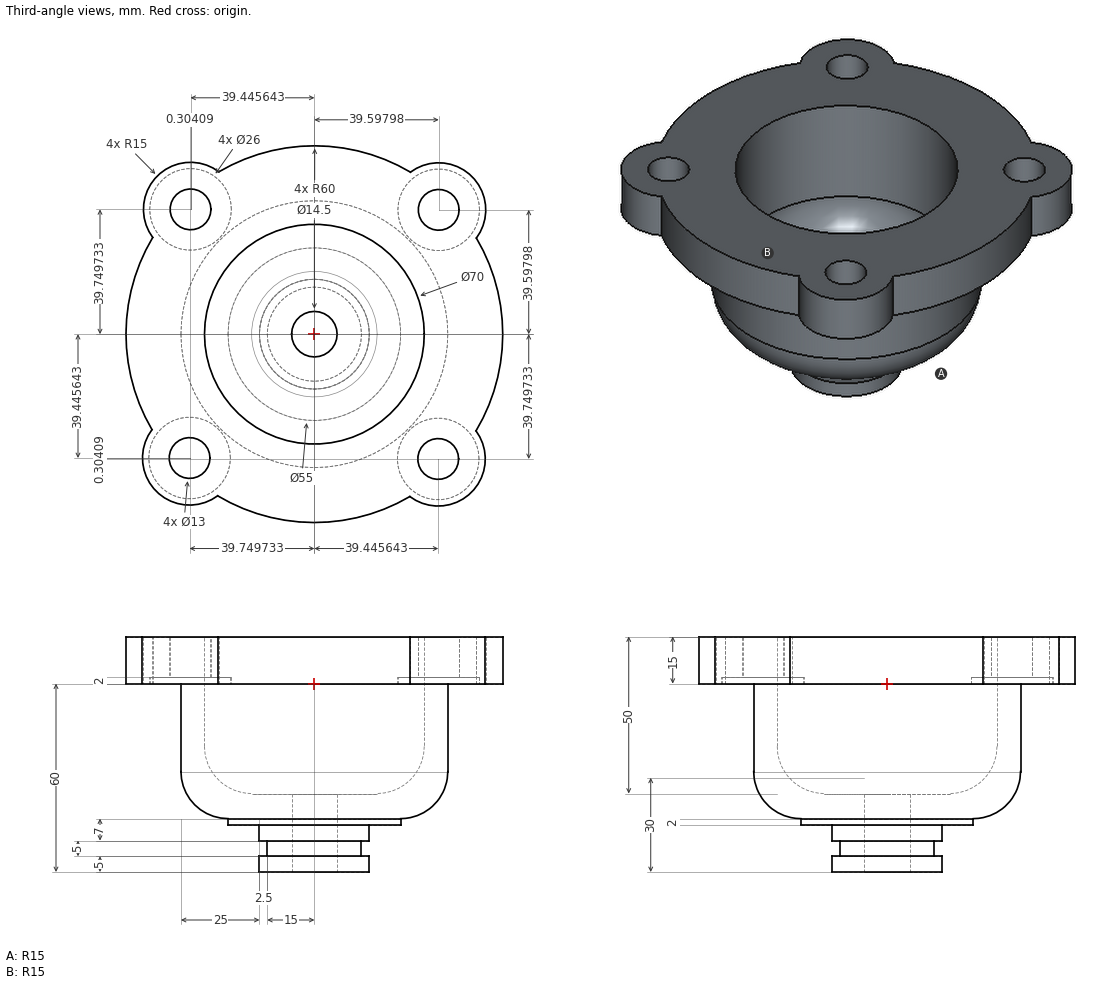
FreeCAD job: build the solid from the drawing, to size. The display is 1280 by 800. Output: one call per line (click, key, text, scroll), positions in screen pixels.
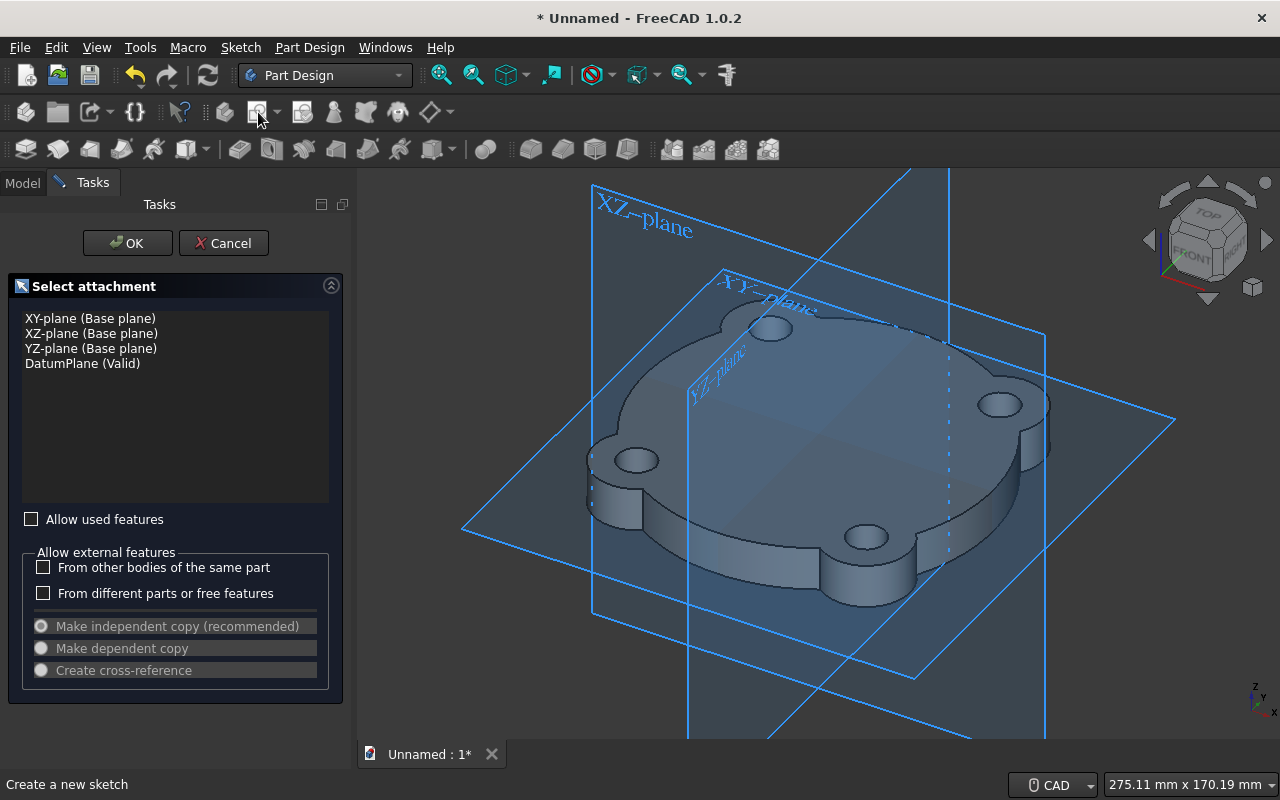
click(82, 334)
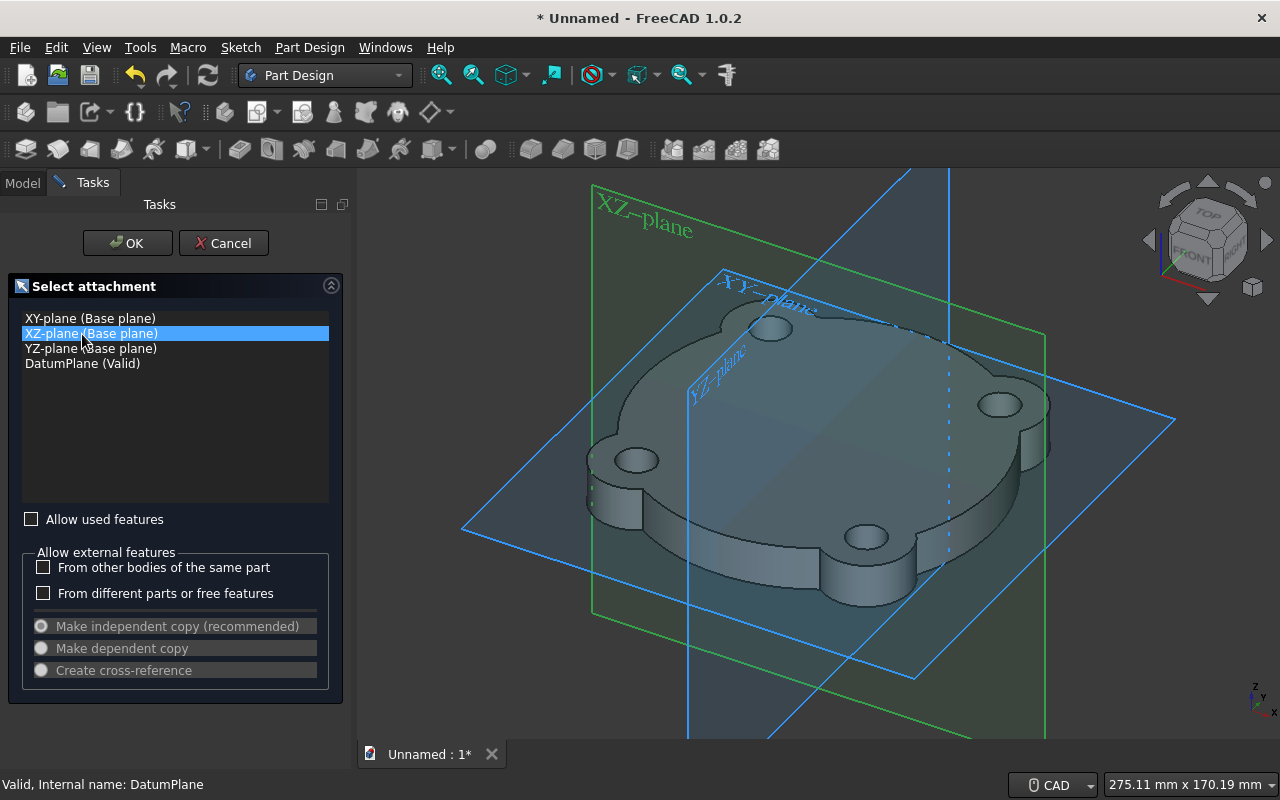
click(128, 243)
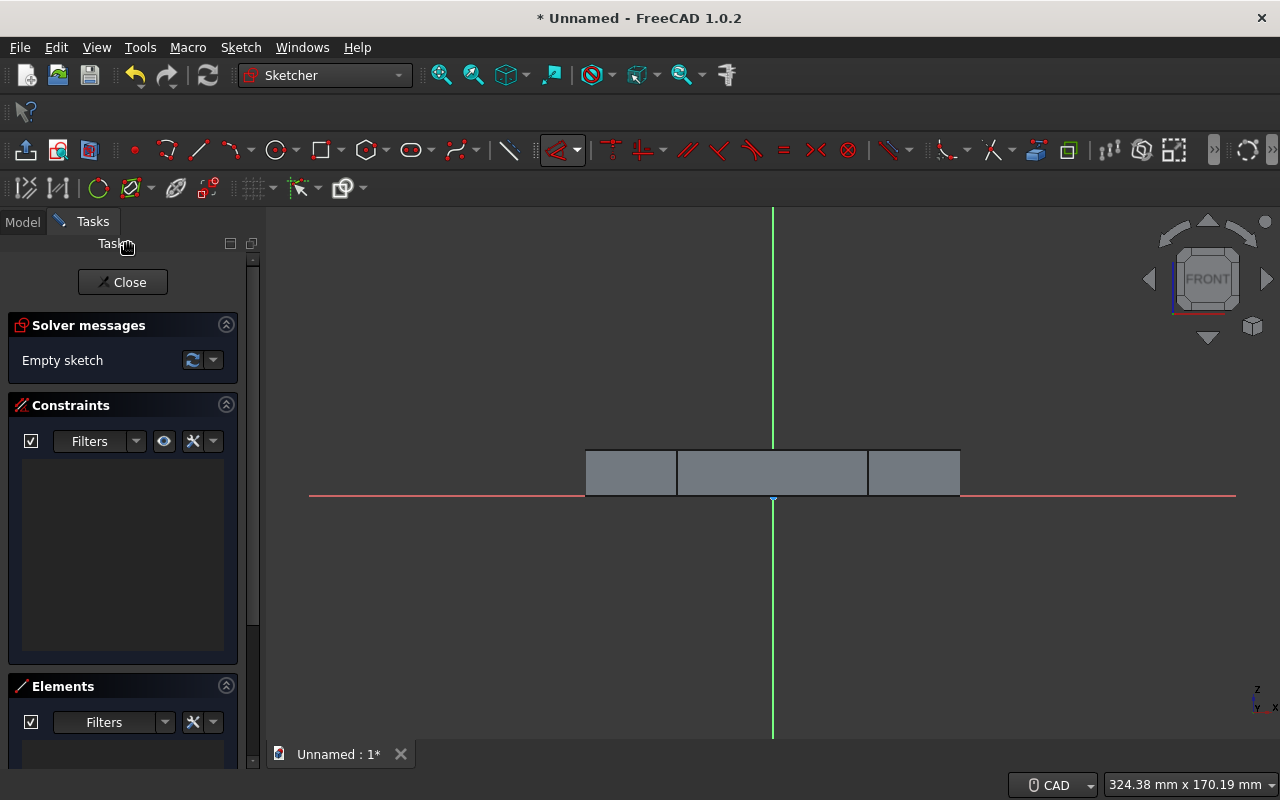
click(90, 150)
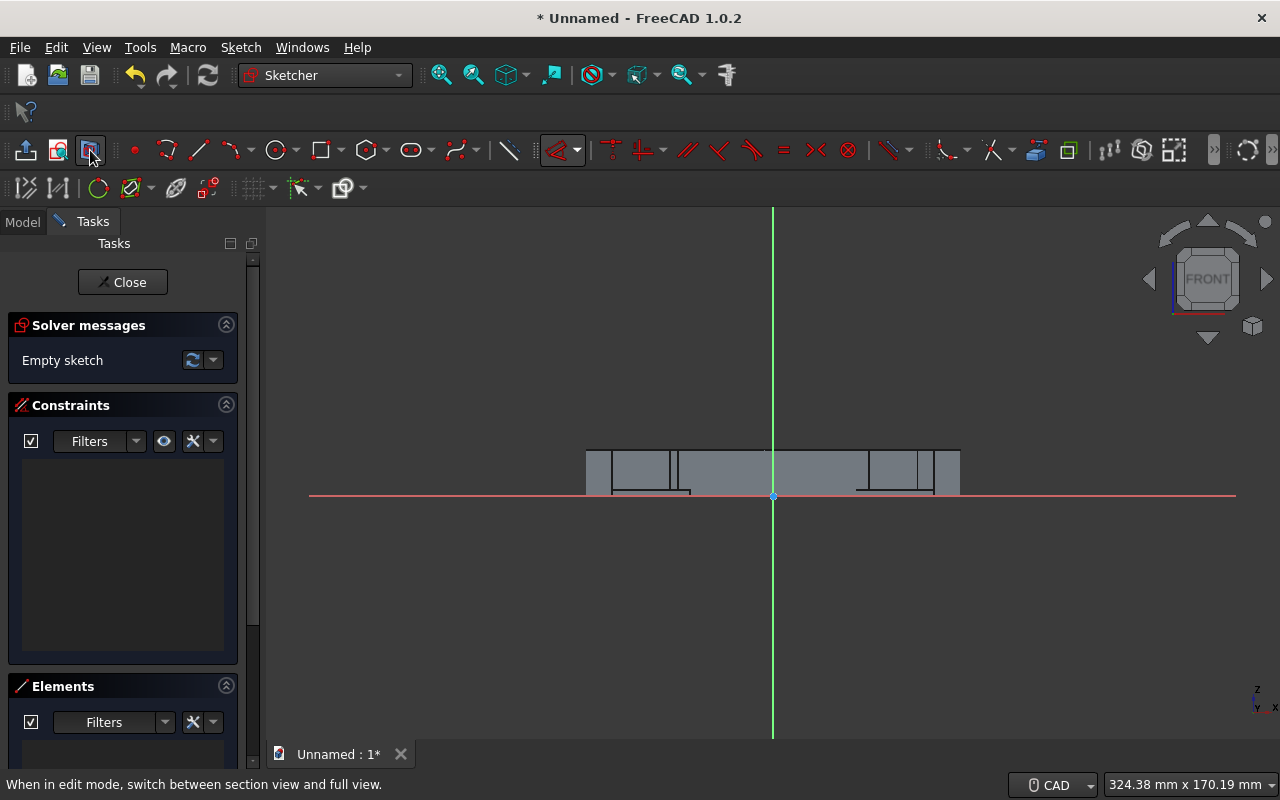
scroll(709, 711, up, 3)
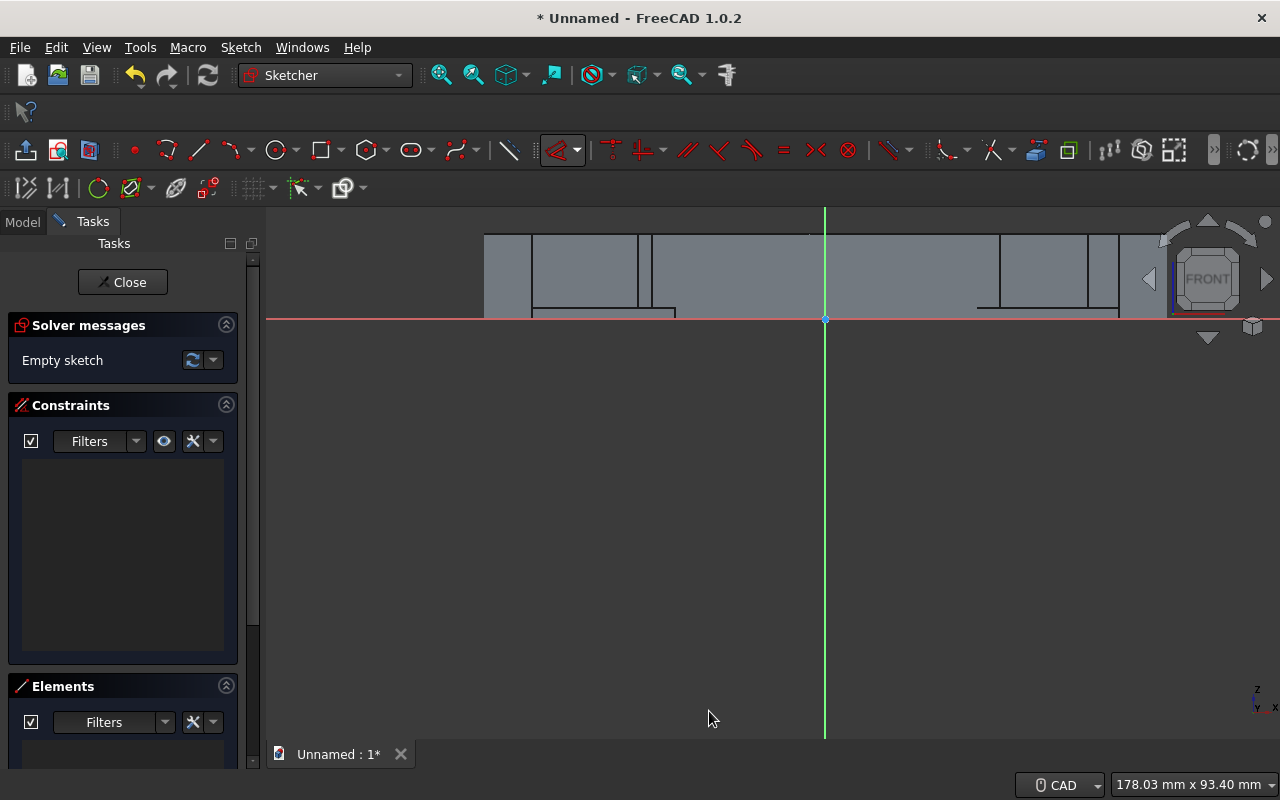
click(168, 150)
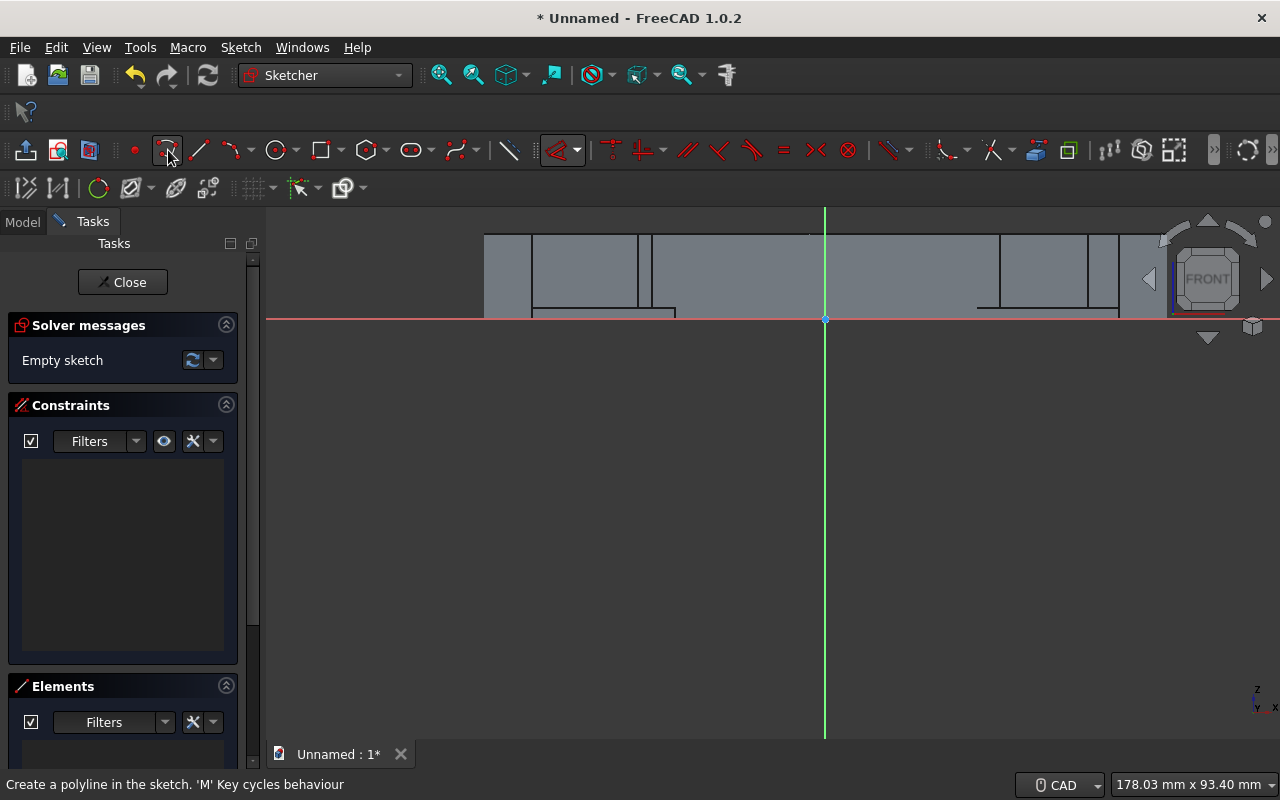
click(825, 319)
click(816, 661)
click(726, 661)
click(726, 633)
click(740, 633)
click(740, 604)
click(726, 604)
click(726, 564)
click(583, 564)
click(583, 328)
click(825, 319)
key(Escape)
key(Escape)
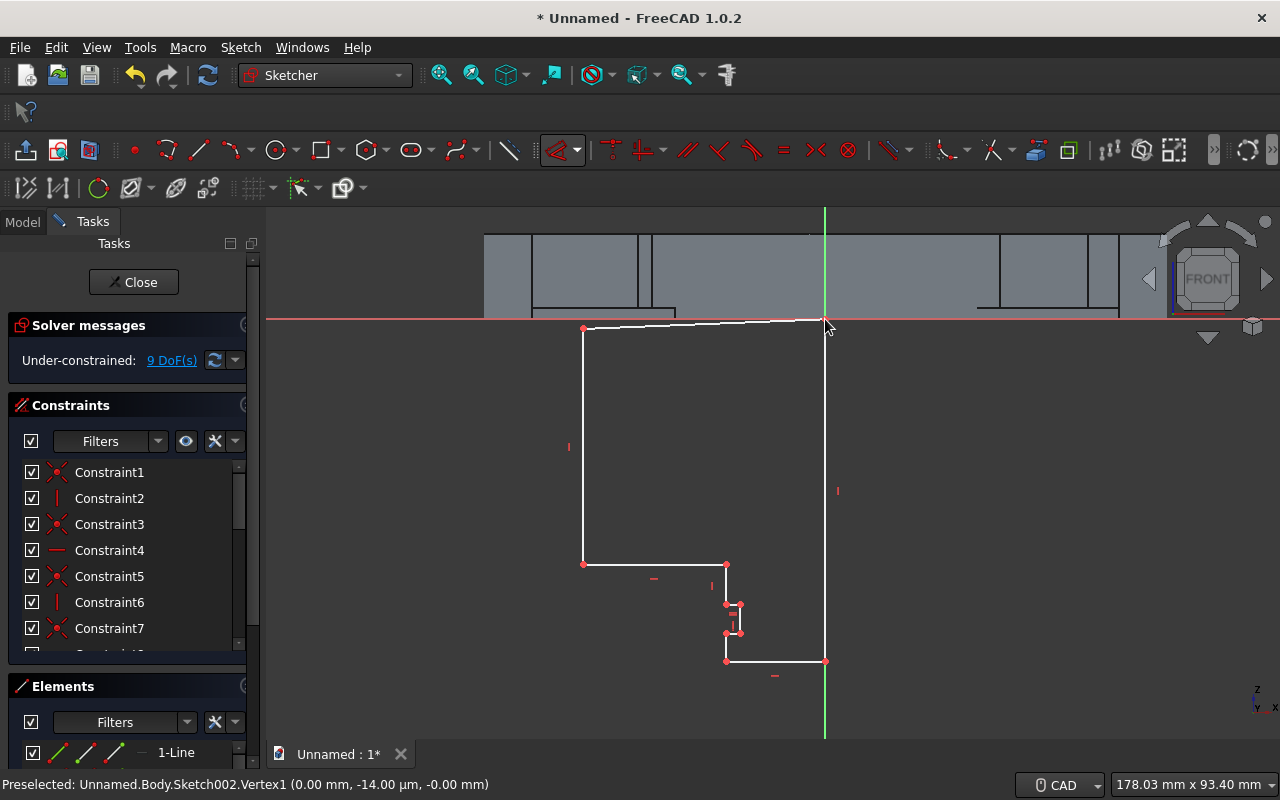
click(753, 322)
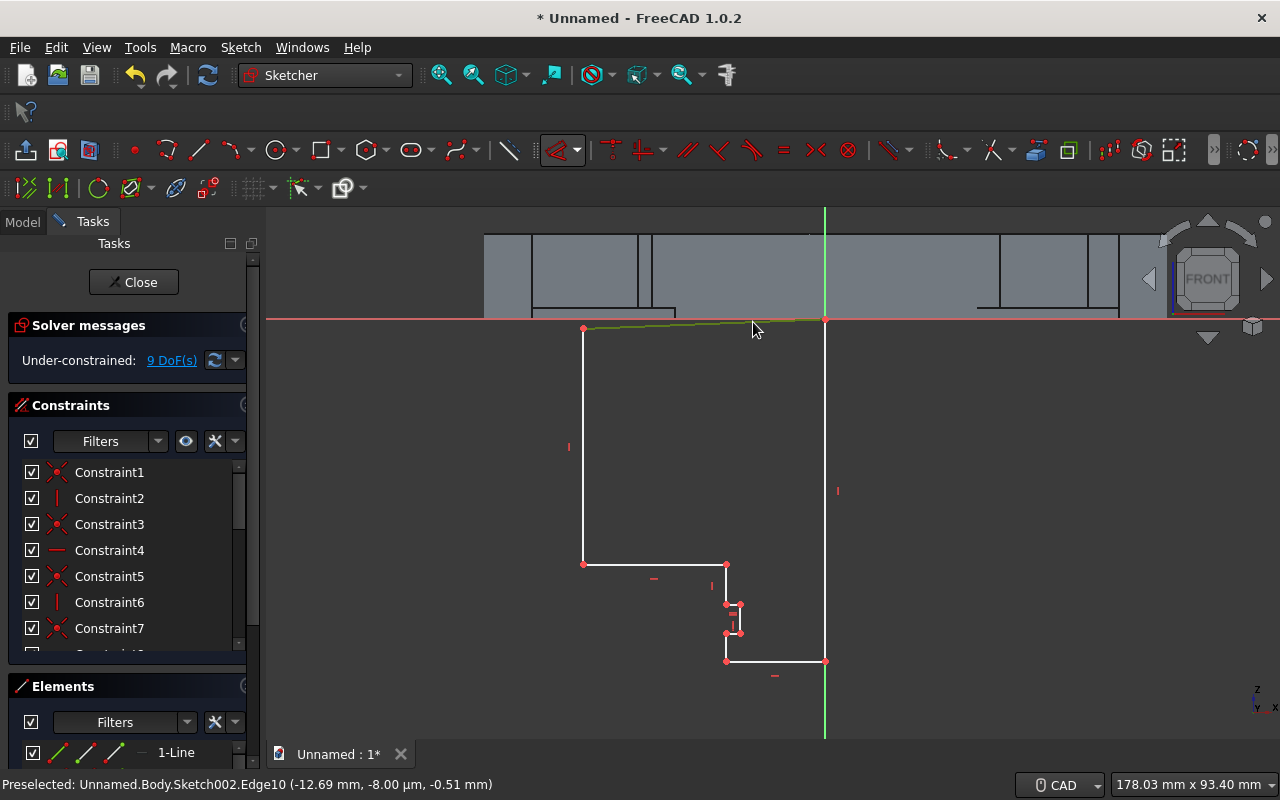
key(h)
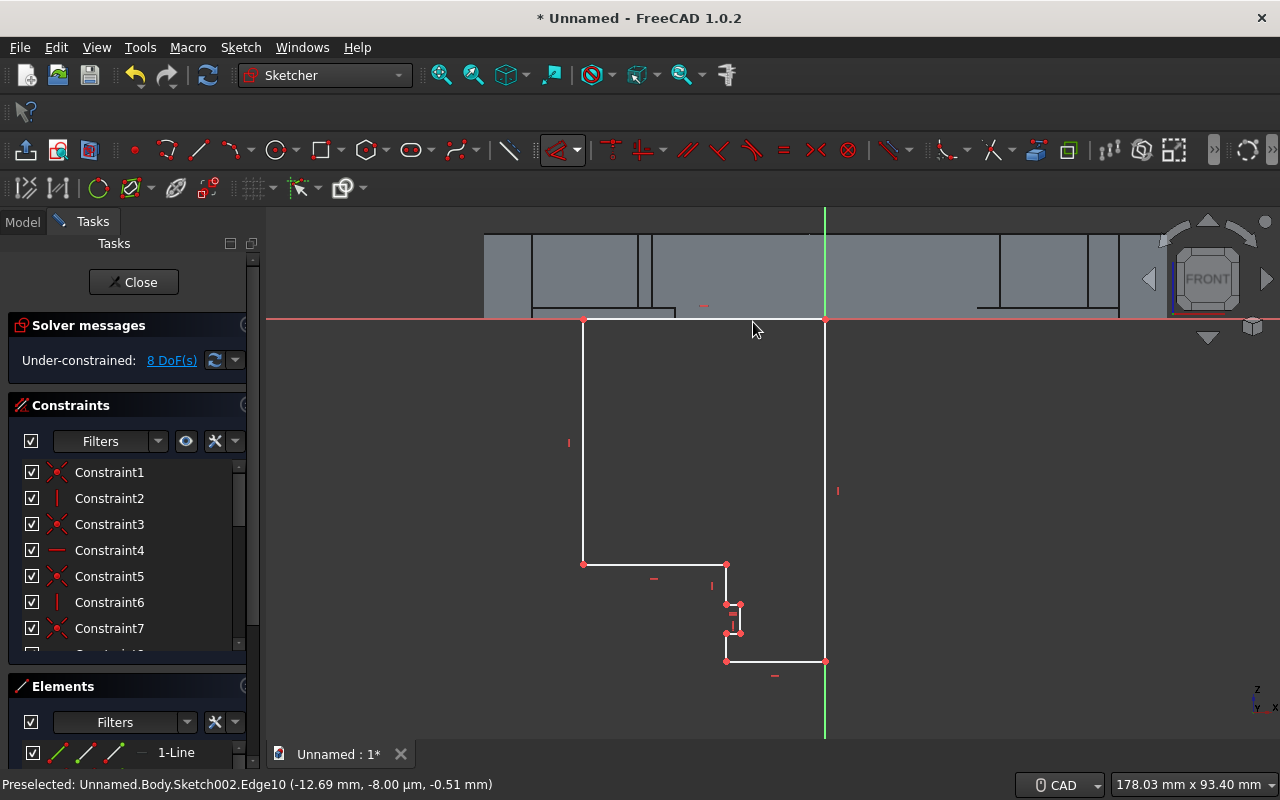
scroll(726, 651, up, 2)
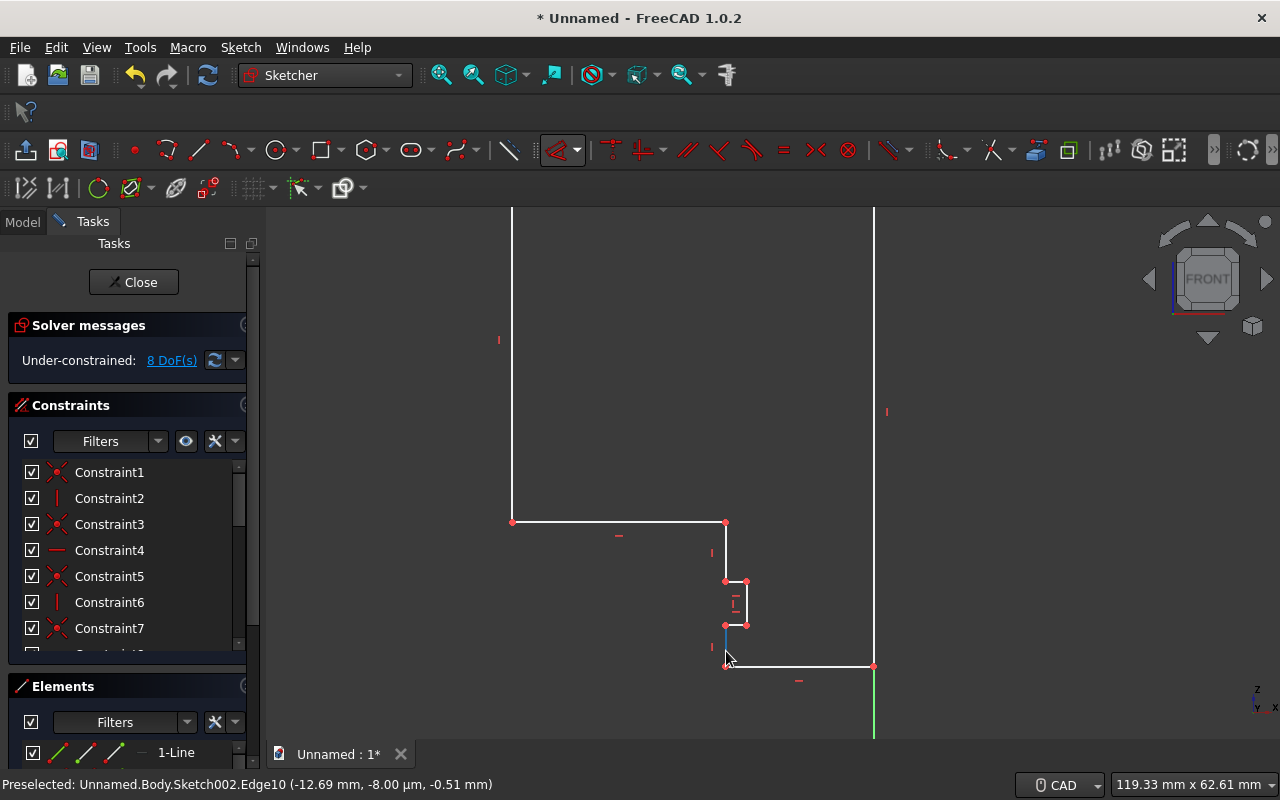
click(726, 650)